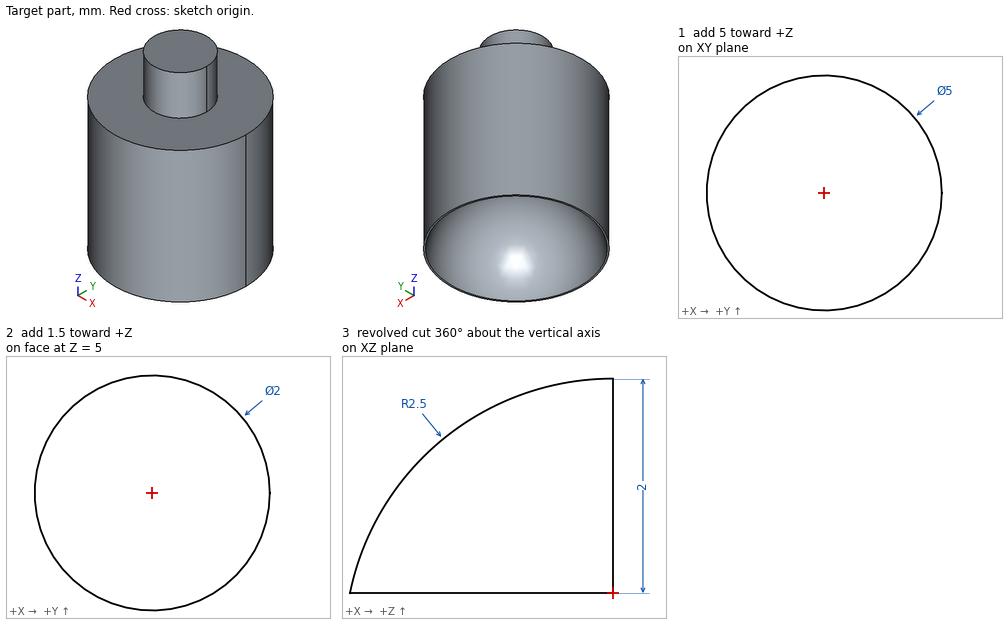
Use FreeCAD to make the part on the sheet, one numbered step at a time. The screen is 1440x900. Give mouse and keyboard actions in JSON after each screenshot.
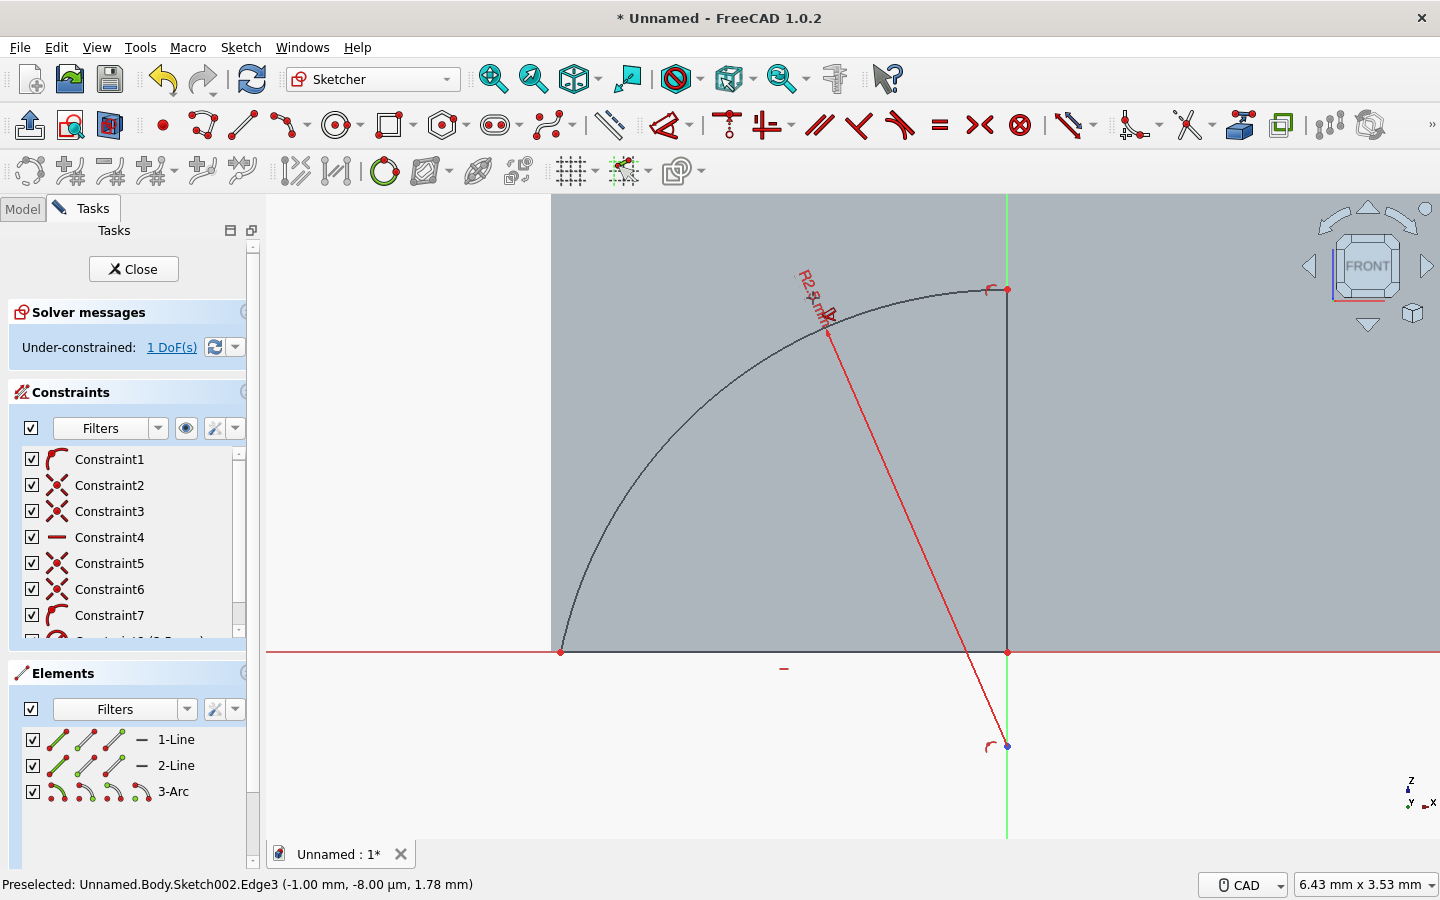
{"action": "left_click", "coordinate": [1007, 398]}
{"action": "left_click", "coordinate": [1041, 471]}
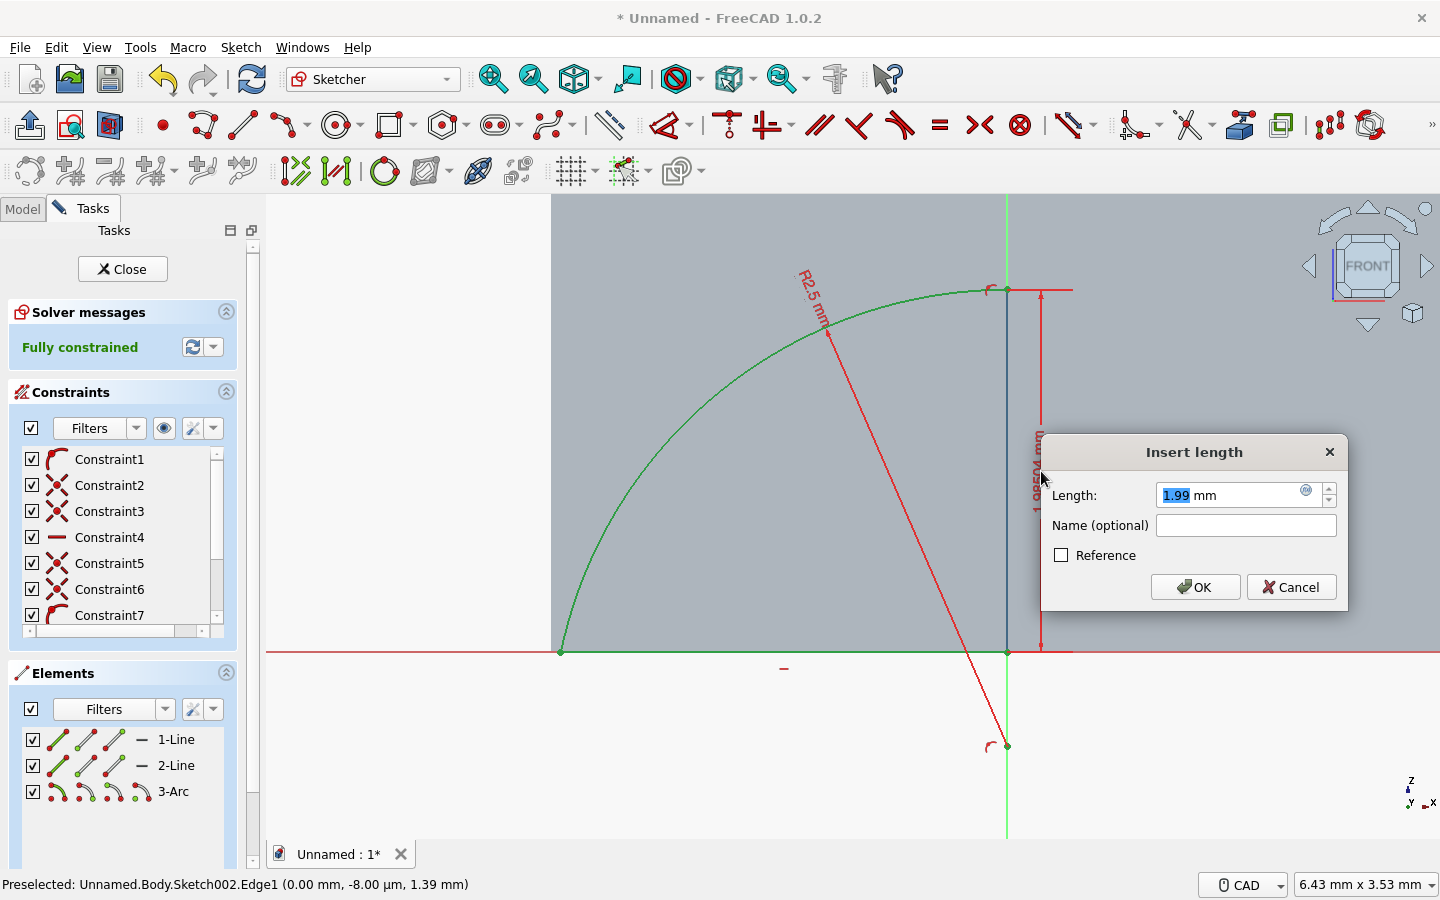
{"action": "type", "text": "2"}
{"action": "key", "text": "Return"}
{"action": "key", "text": "Escape"}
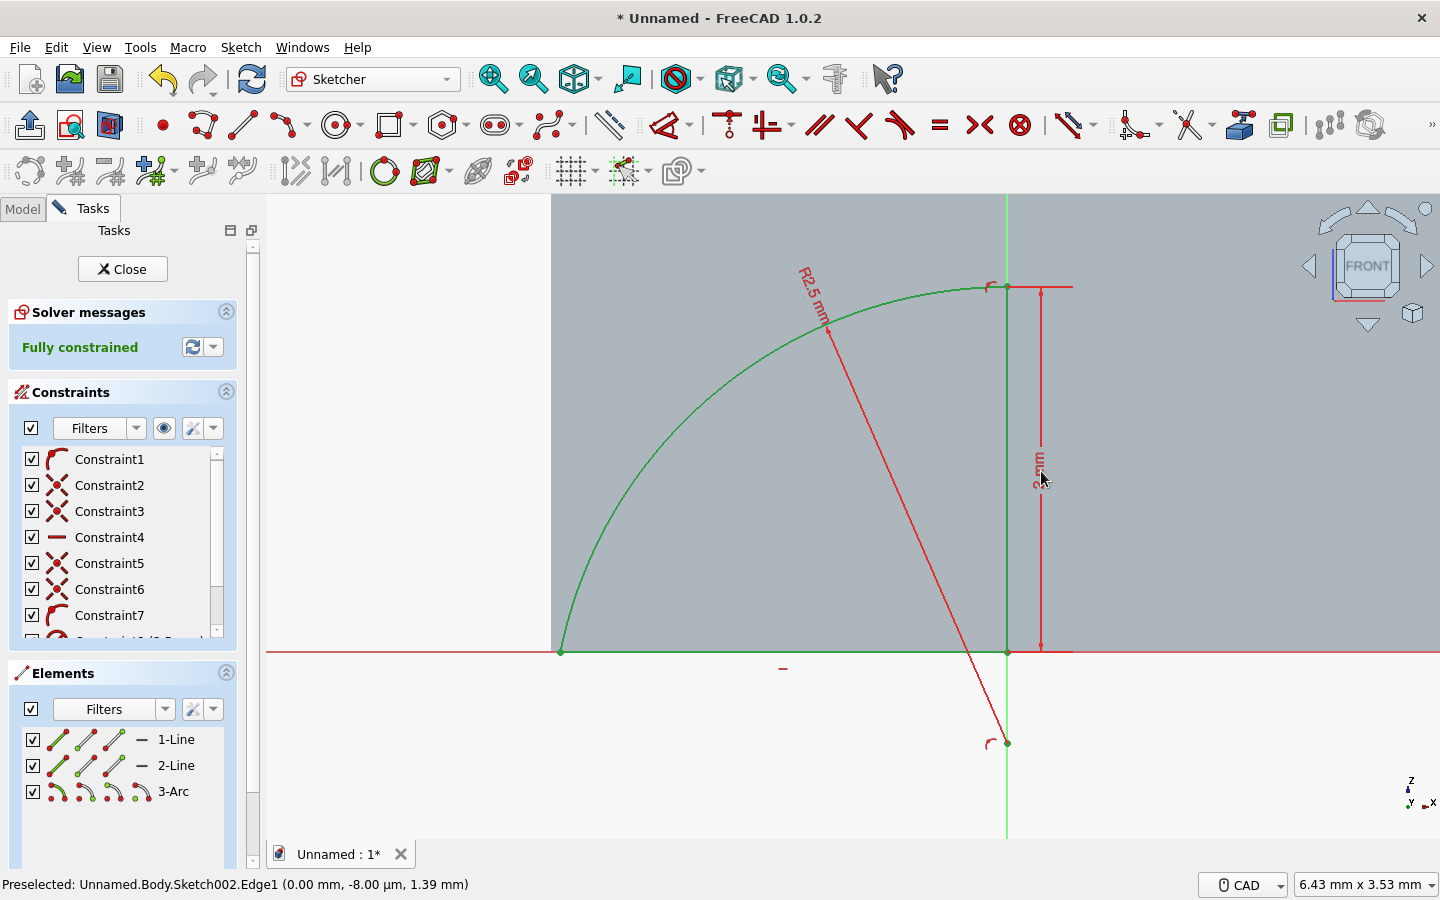
{"action": "left_click", "coordinate": [123, 269]}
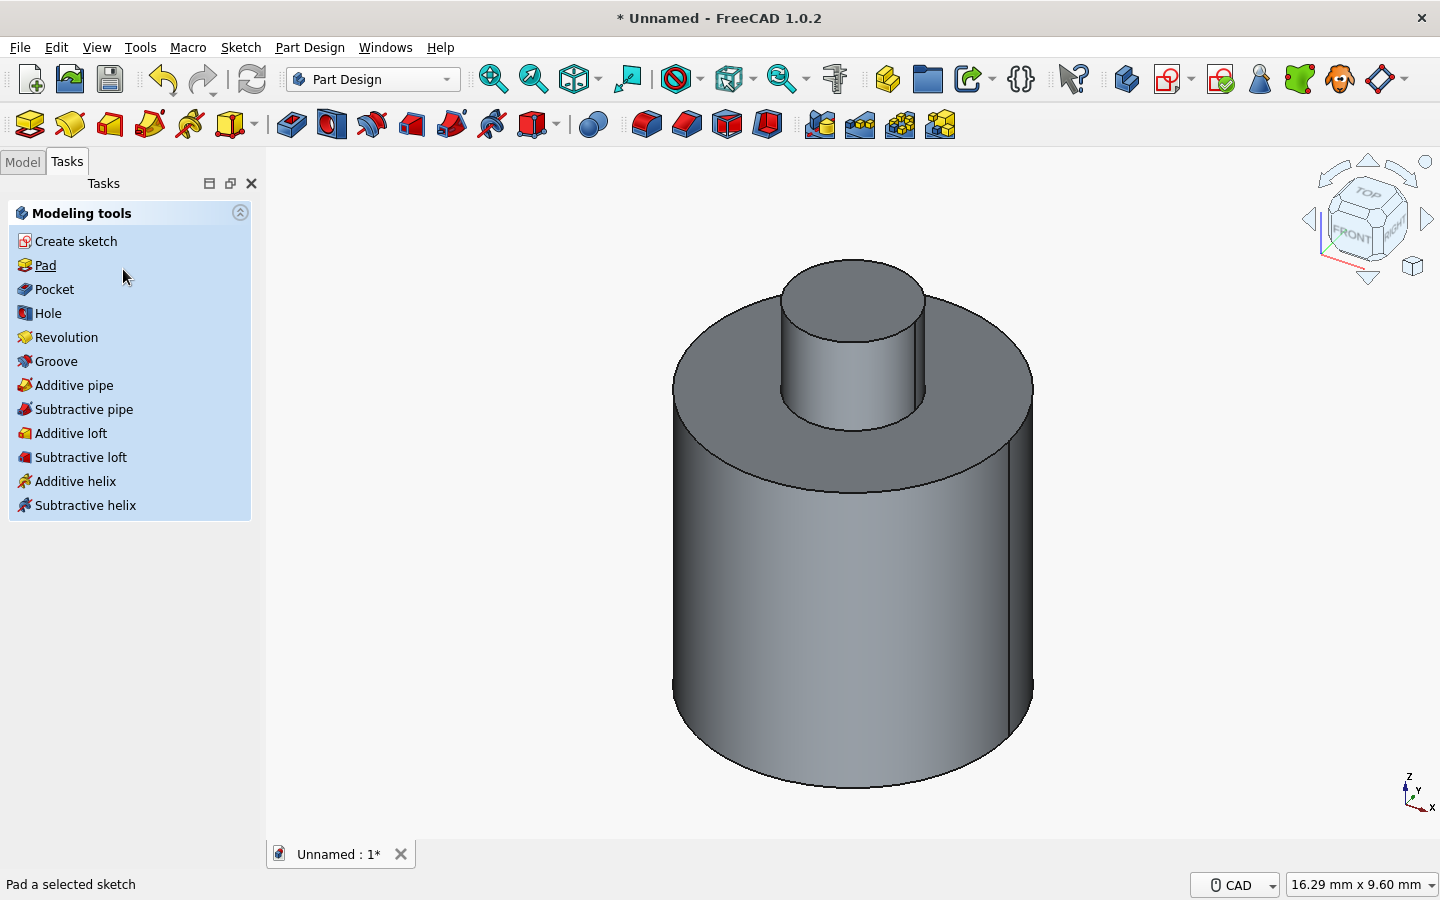
{"action": "left_click", "coordinate": [372, 124]}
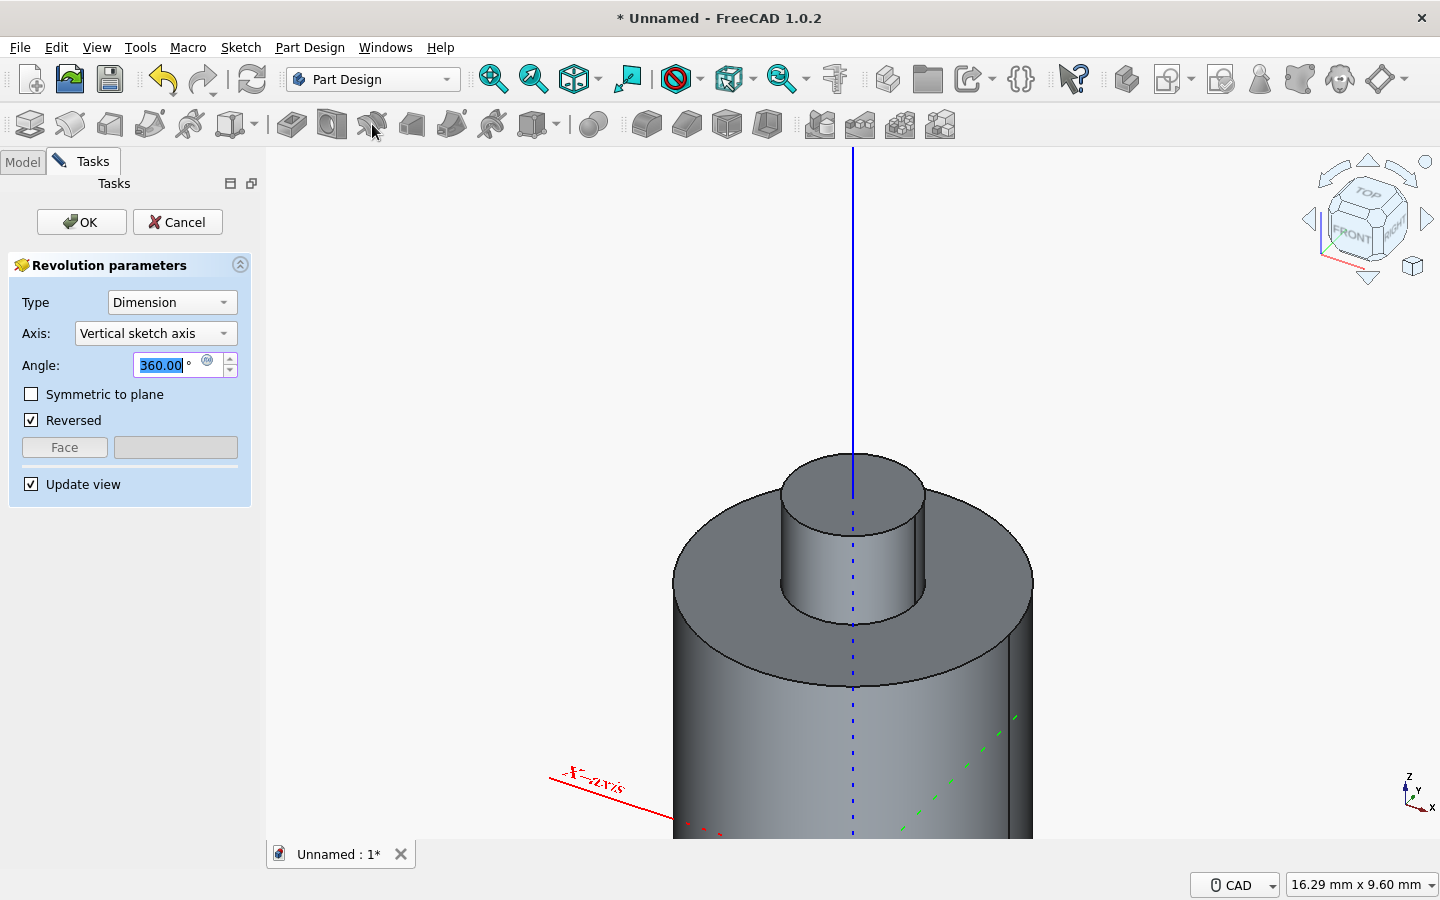
{"action": "left_click", "coordinate": [82, 222]}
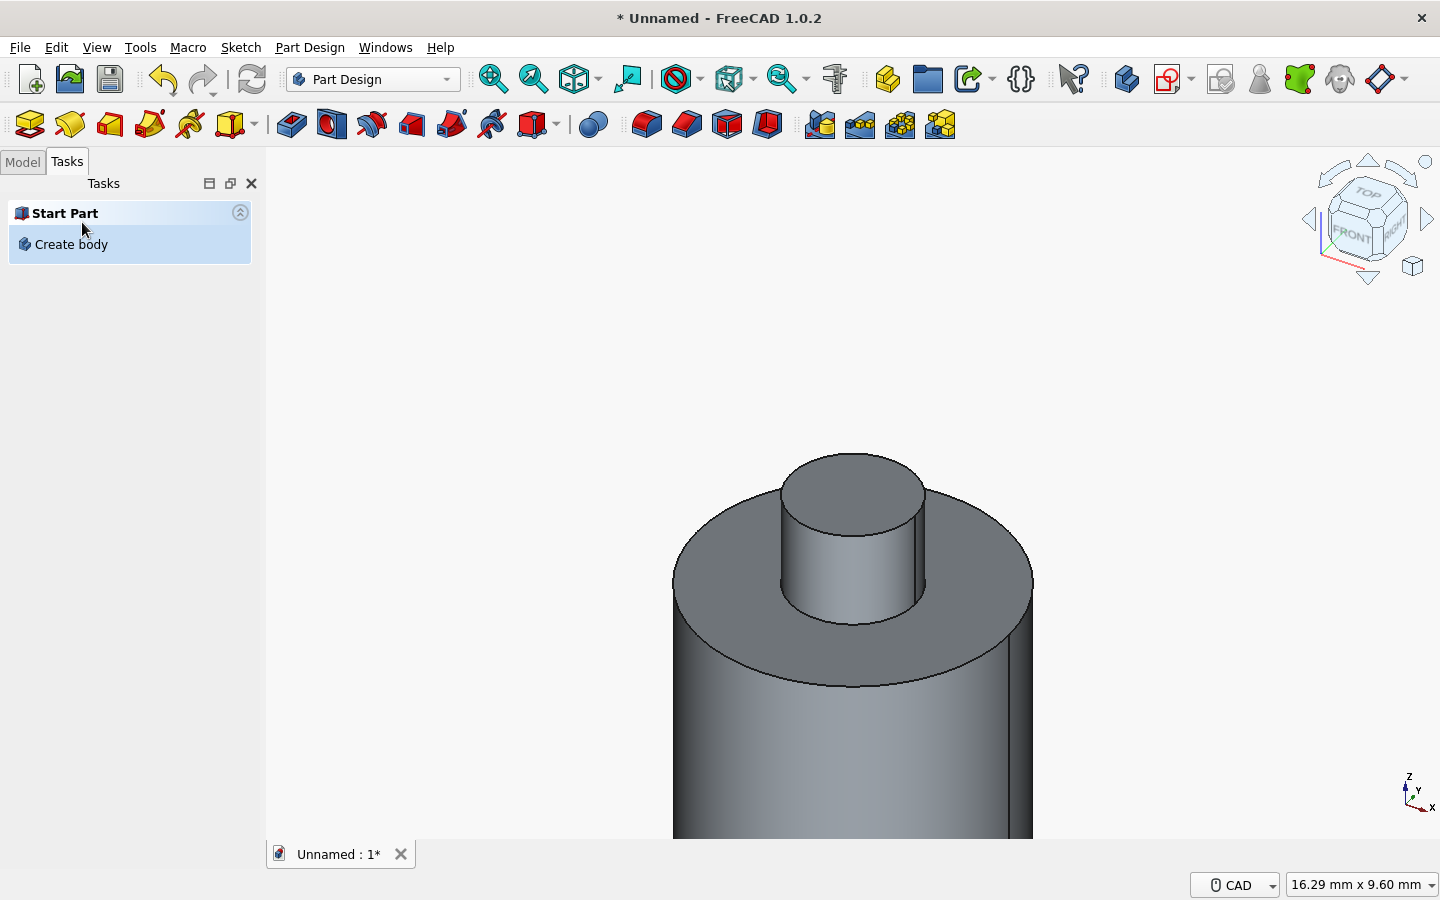
{"action": "key", "text": "0"}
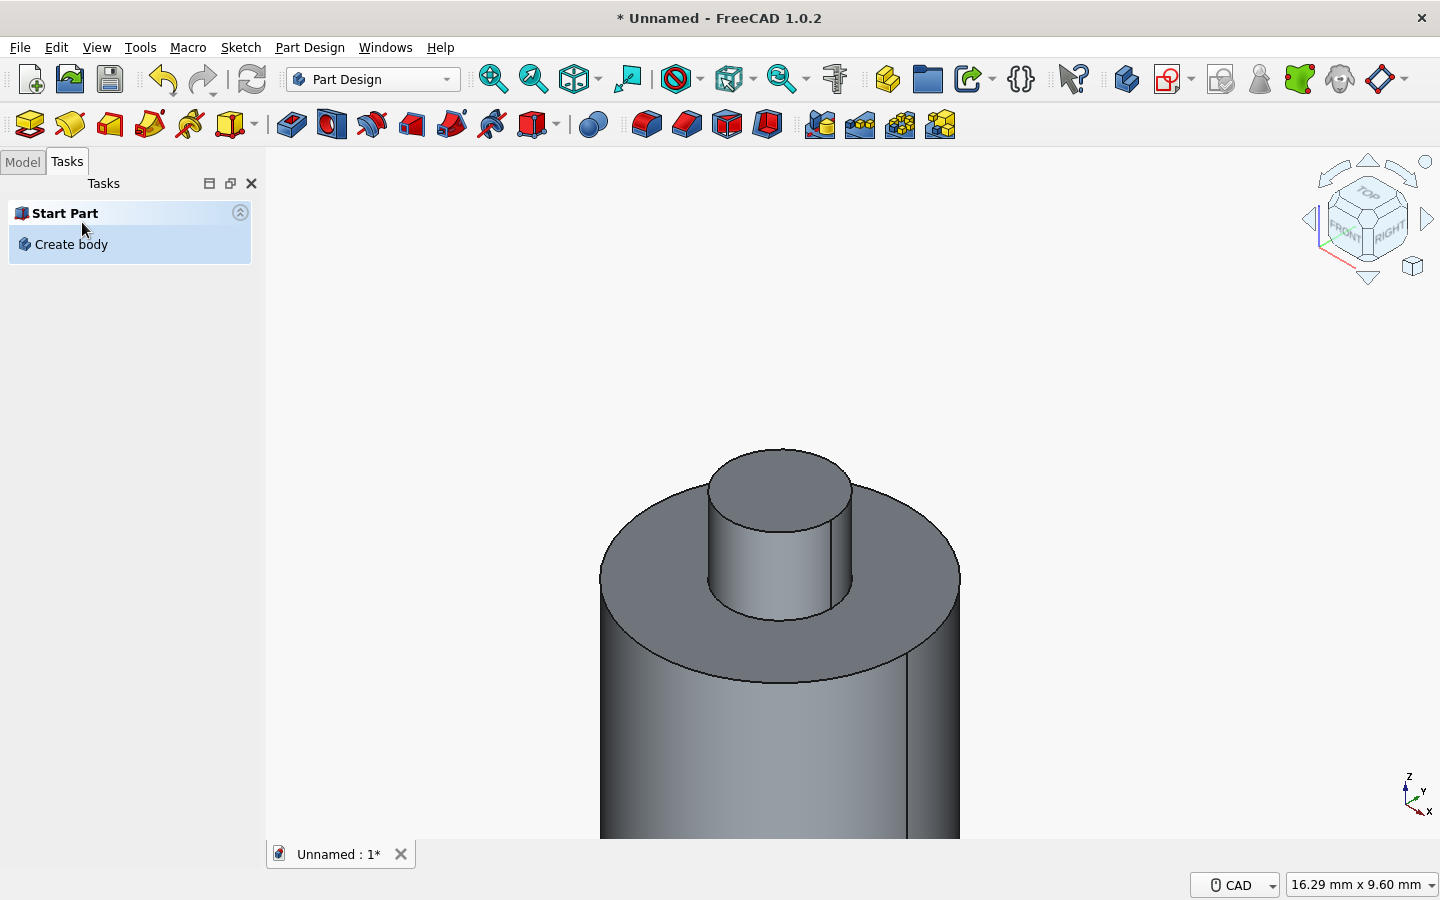
{"action": "left_click", "coordinate": [494, 80]}